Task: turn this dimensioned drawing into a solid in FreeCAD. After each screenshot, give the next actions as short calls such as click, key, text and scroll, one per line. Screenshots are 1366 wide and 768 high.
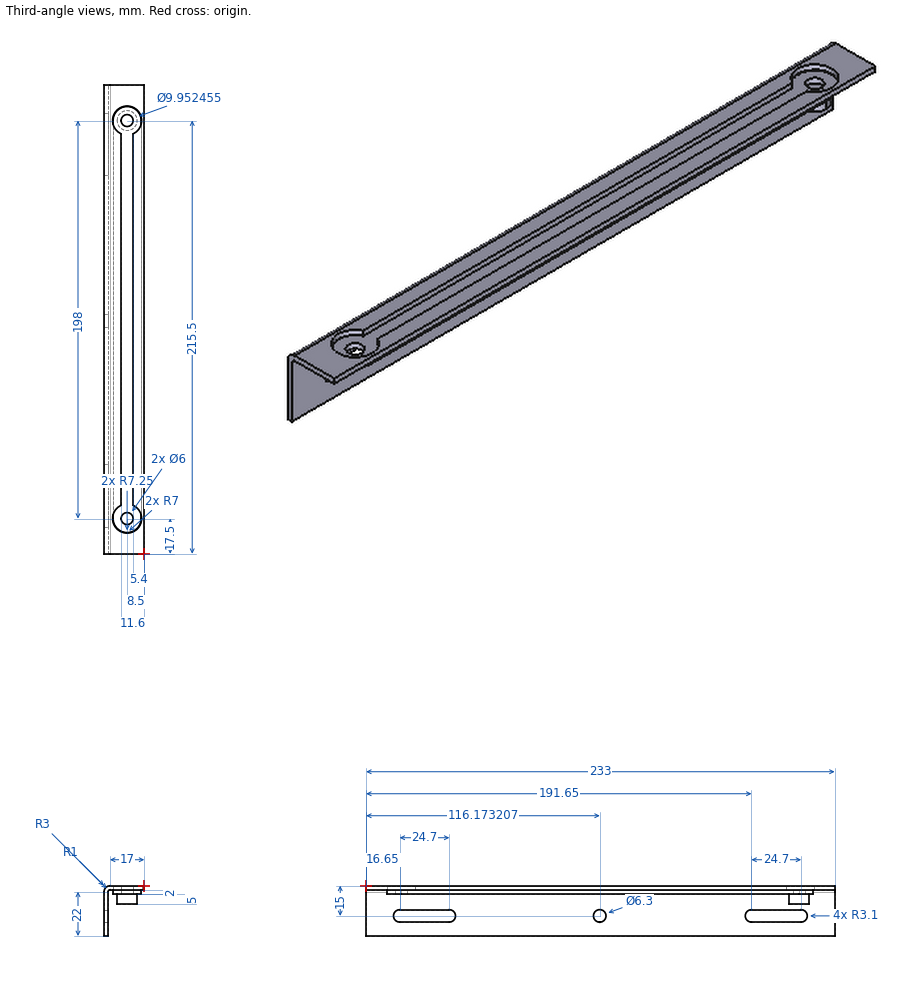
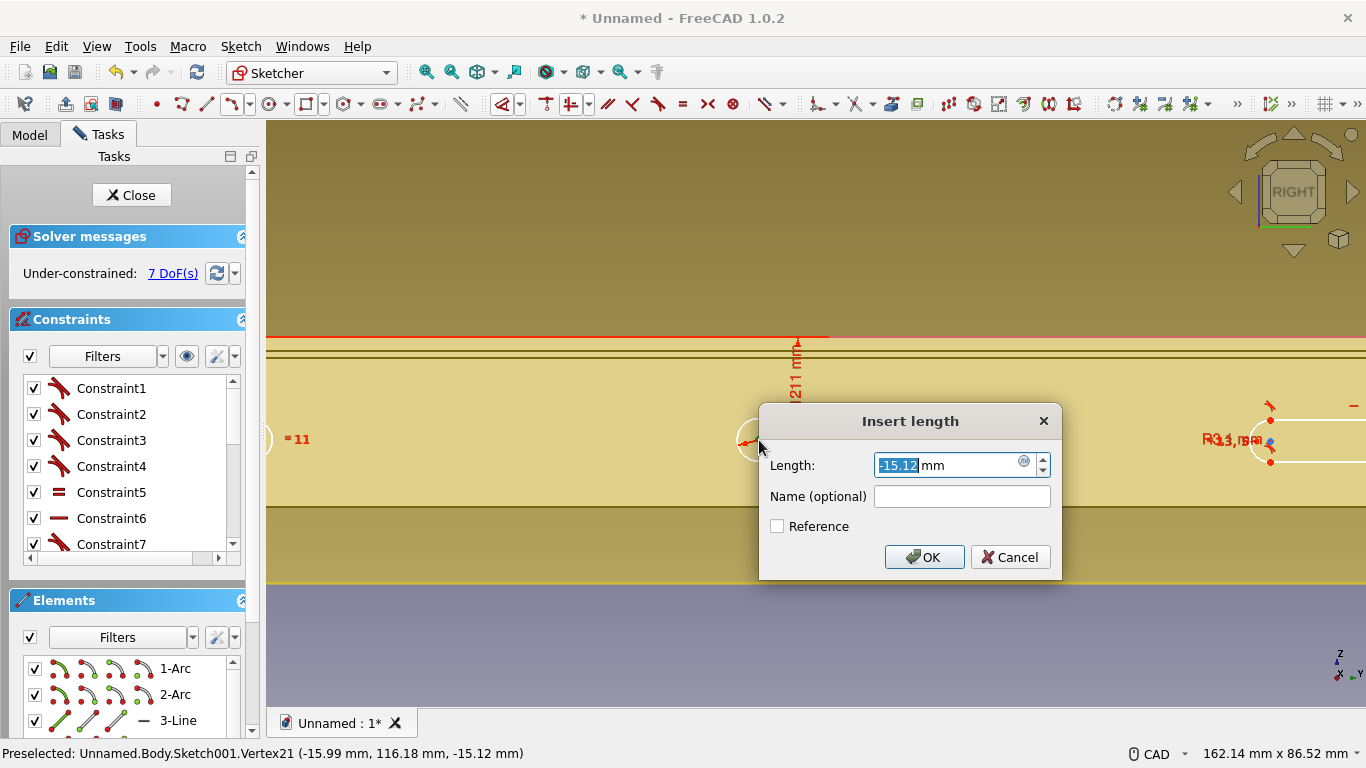
text(-15)
key(Return)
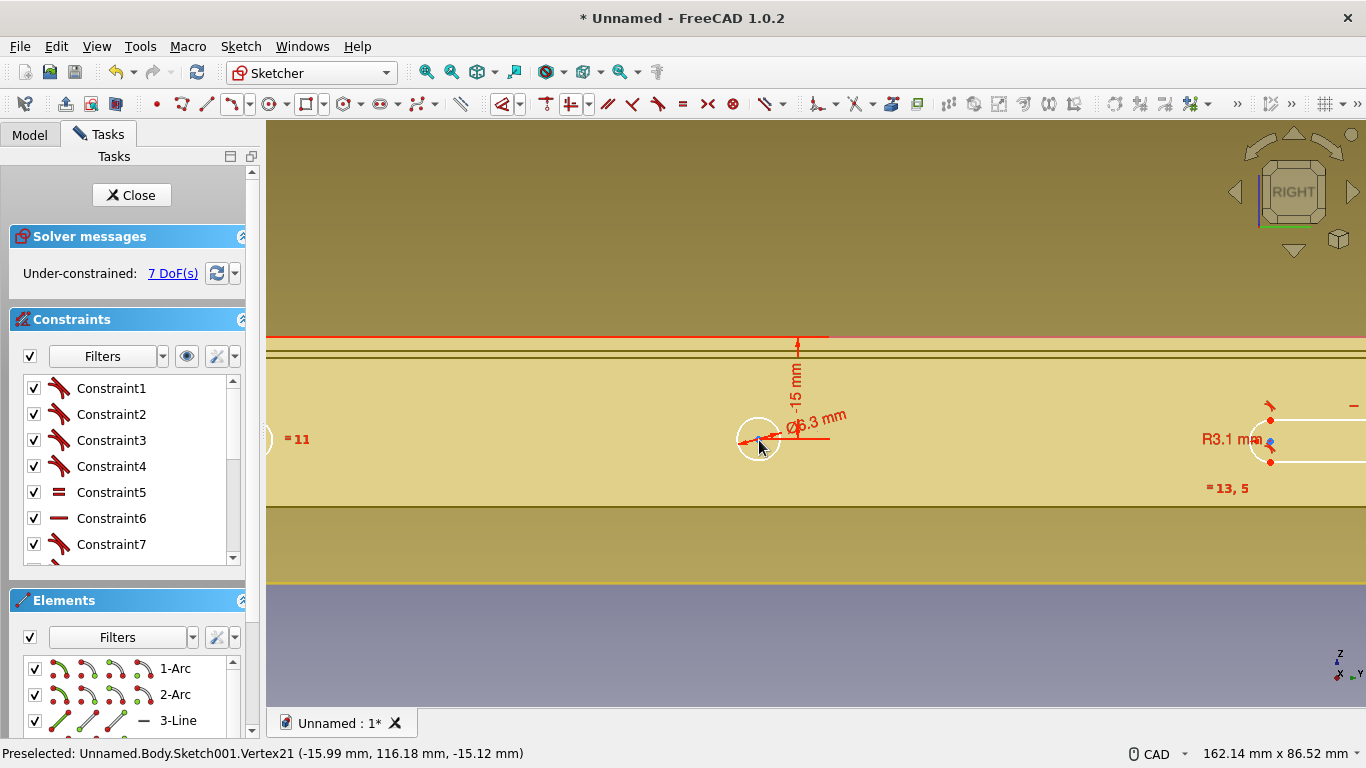
scroll(774, 425, down, 4)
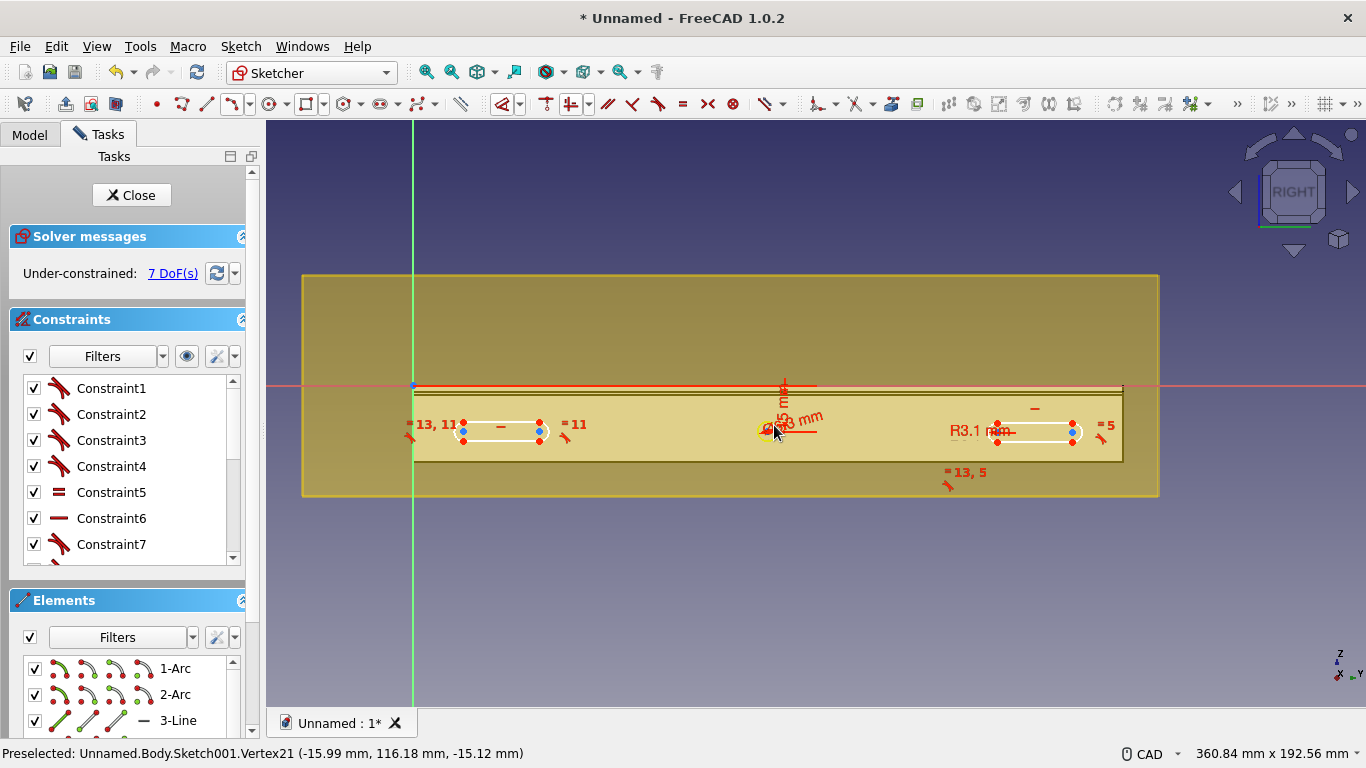
scroll(998, 433, up, 2)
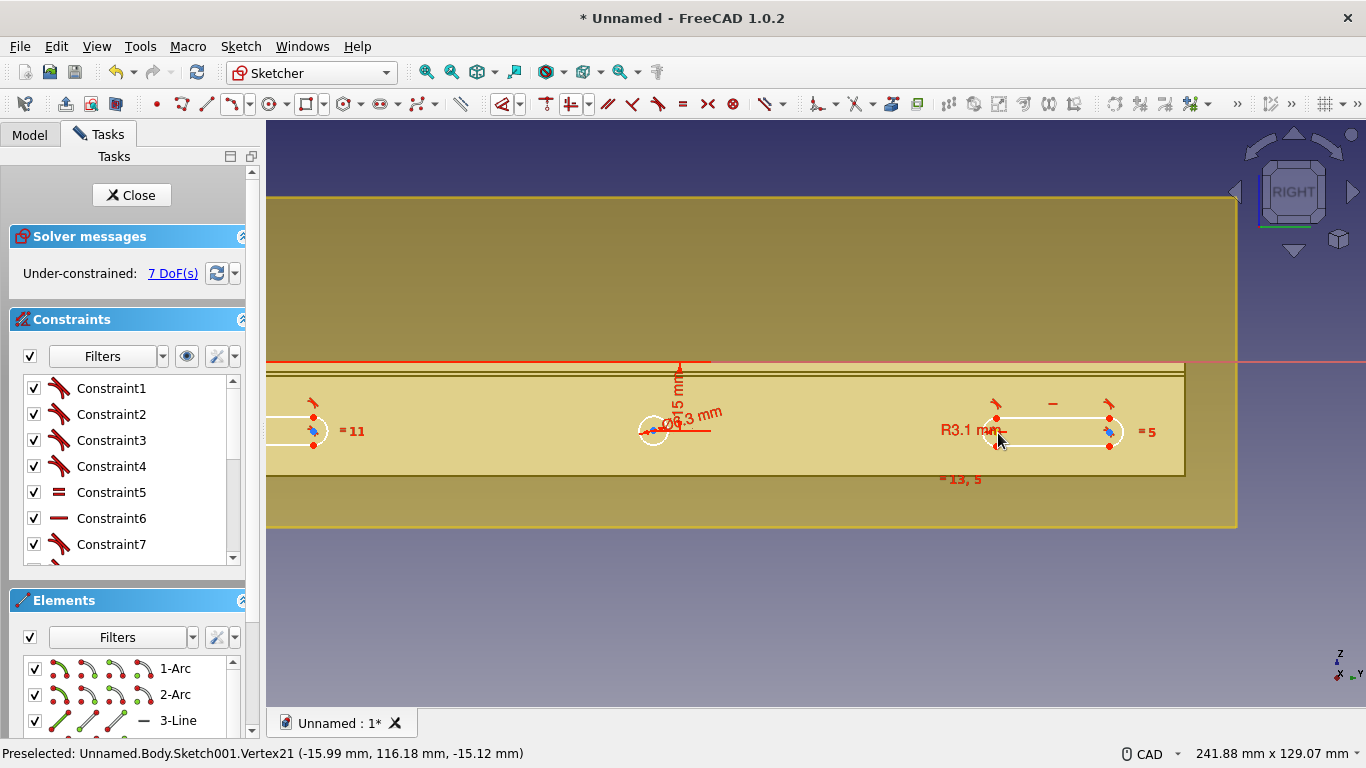
click(997, 432)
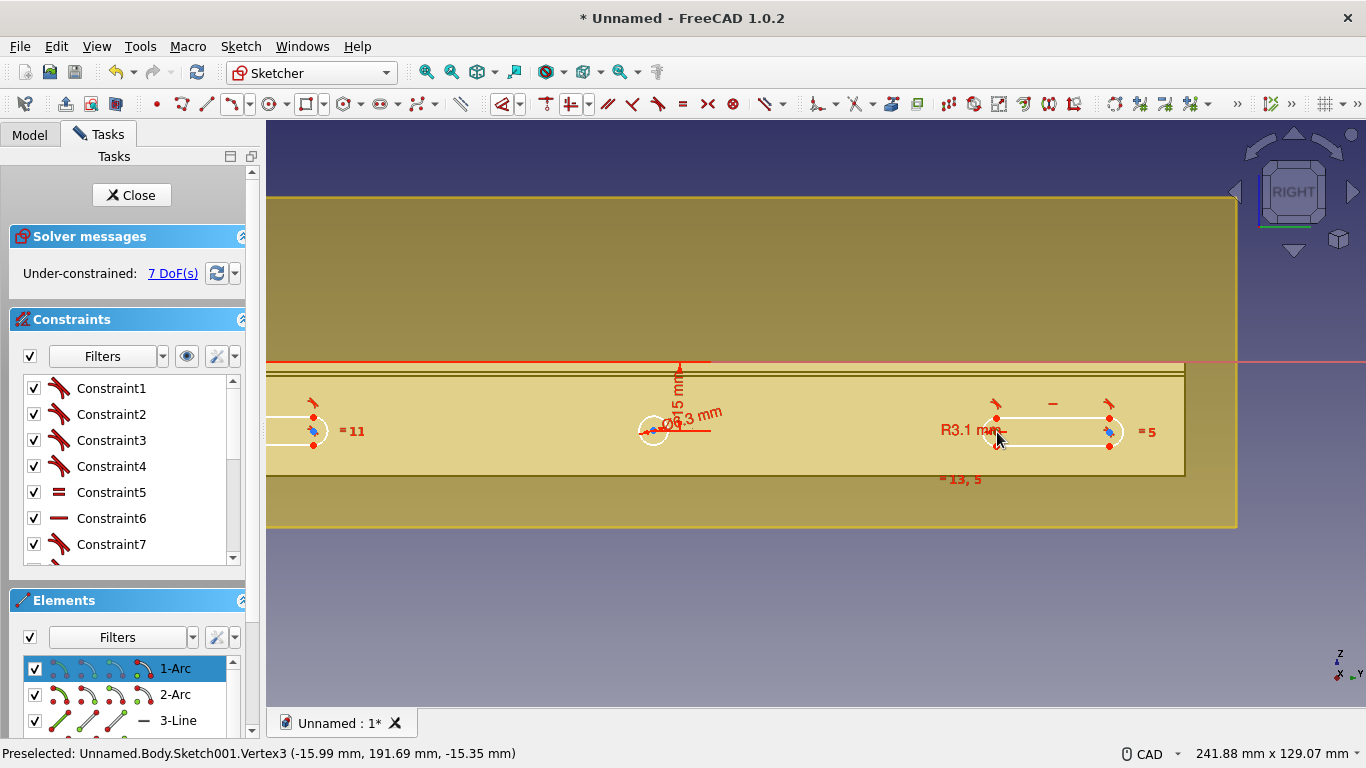
click(520, 104)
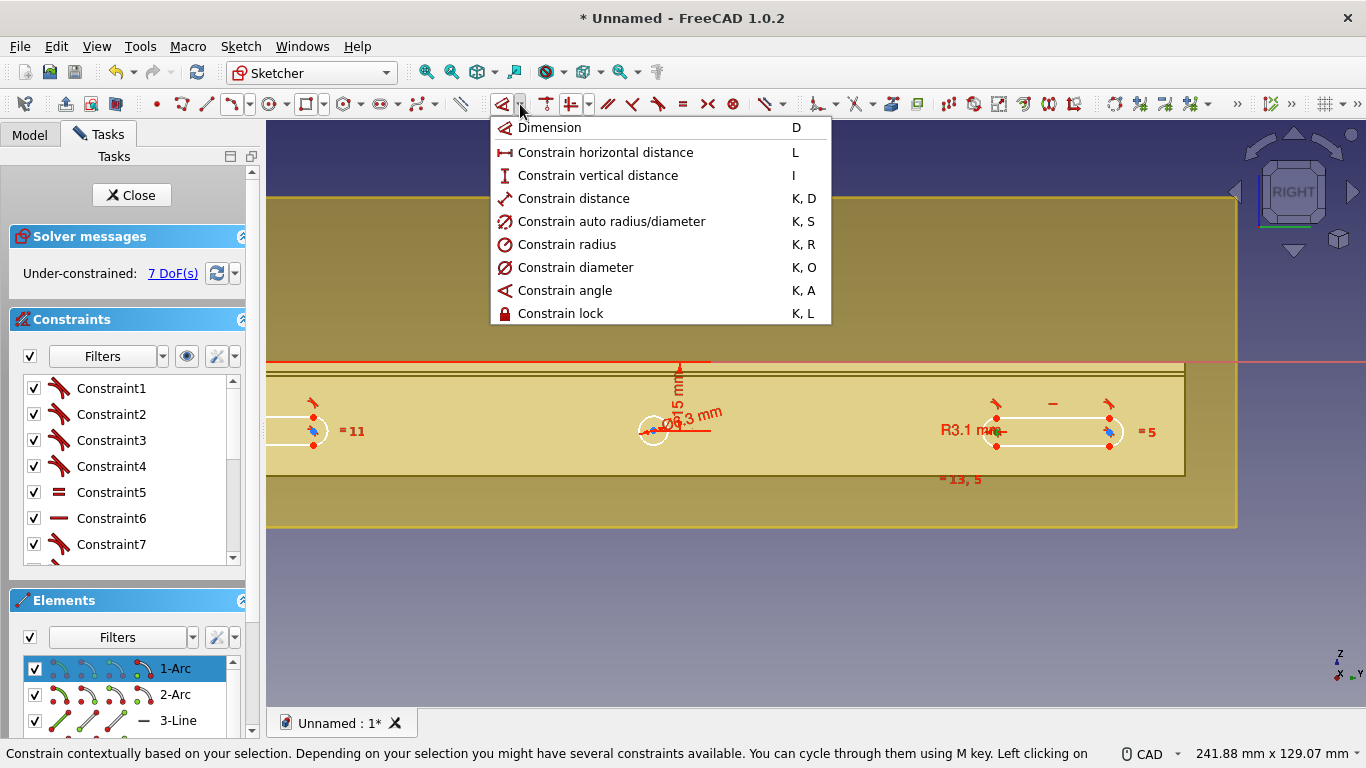
click(661, 176)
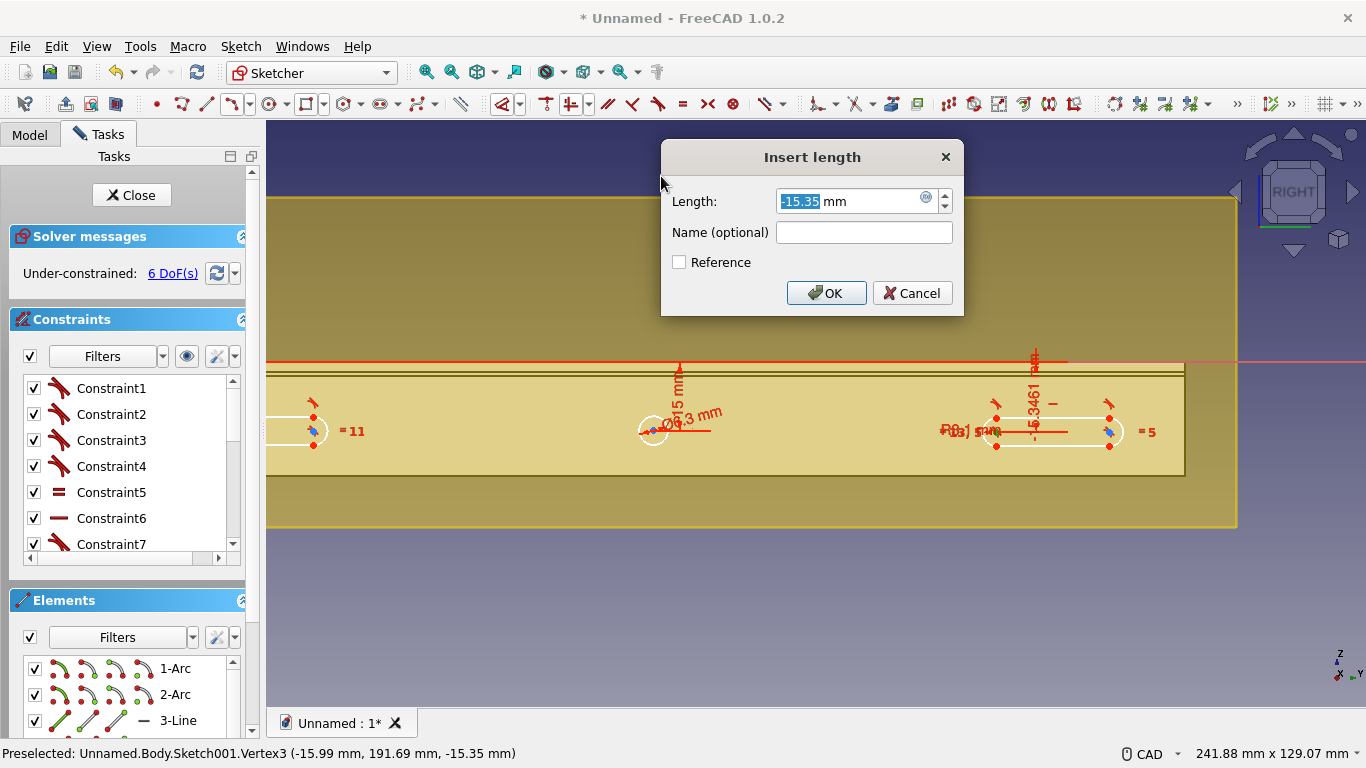
text(-15)
key(Return)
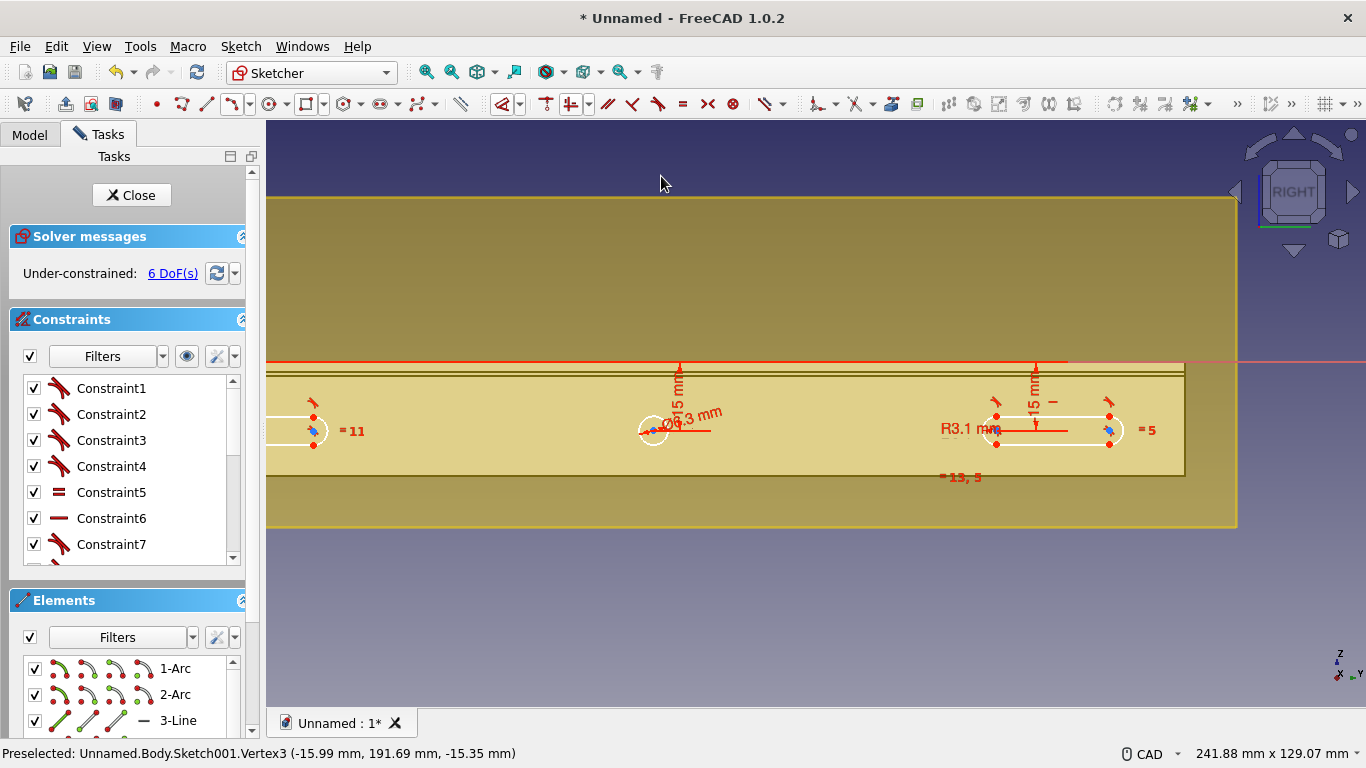
scroll(998, 433, down, 2)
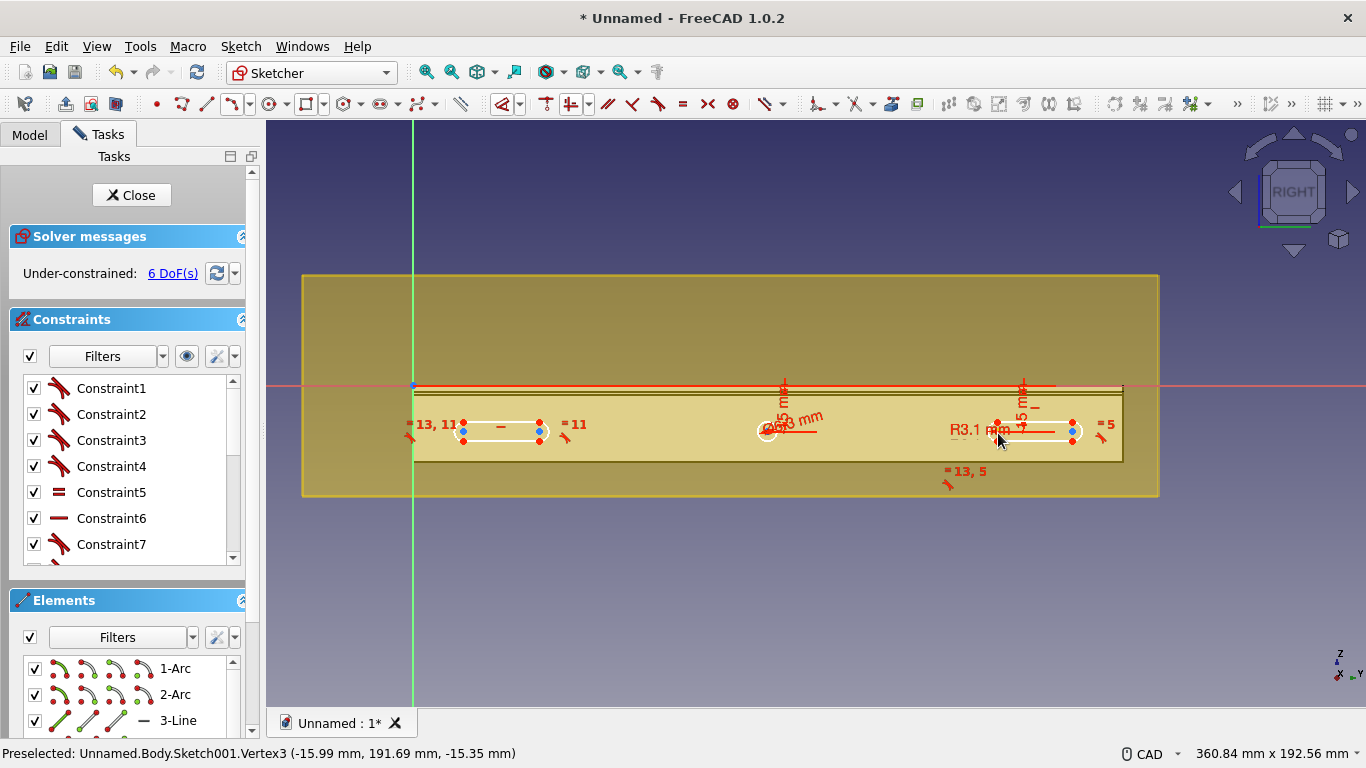
scroll(464, 432, up, 2)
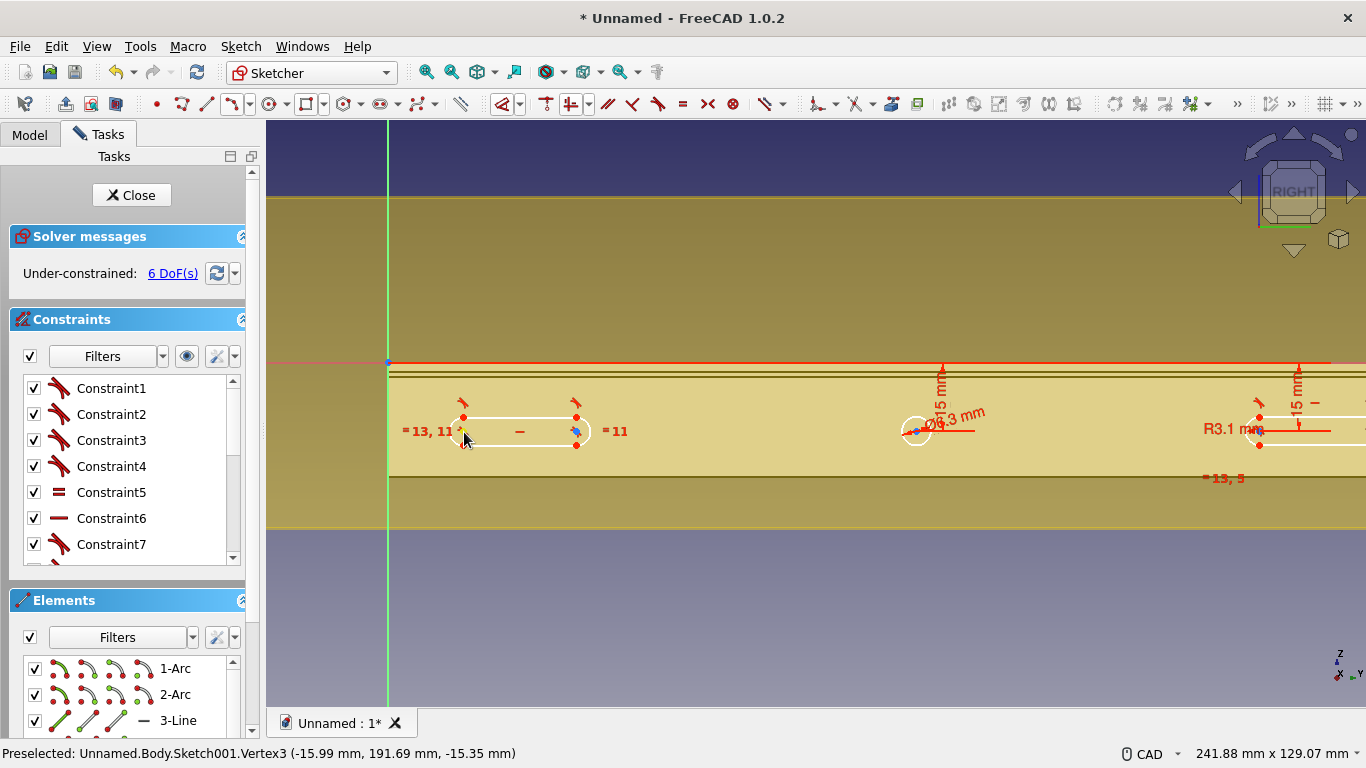
click(464, 432)